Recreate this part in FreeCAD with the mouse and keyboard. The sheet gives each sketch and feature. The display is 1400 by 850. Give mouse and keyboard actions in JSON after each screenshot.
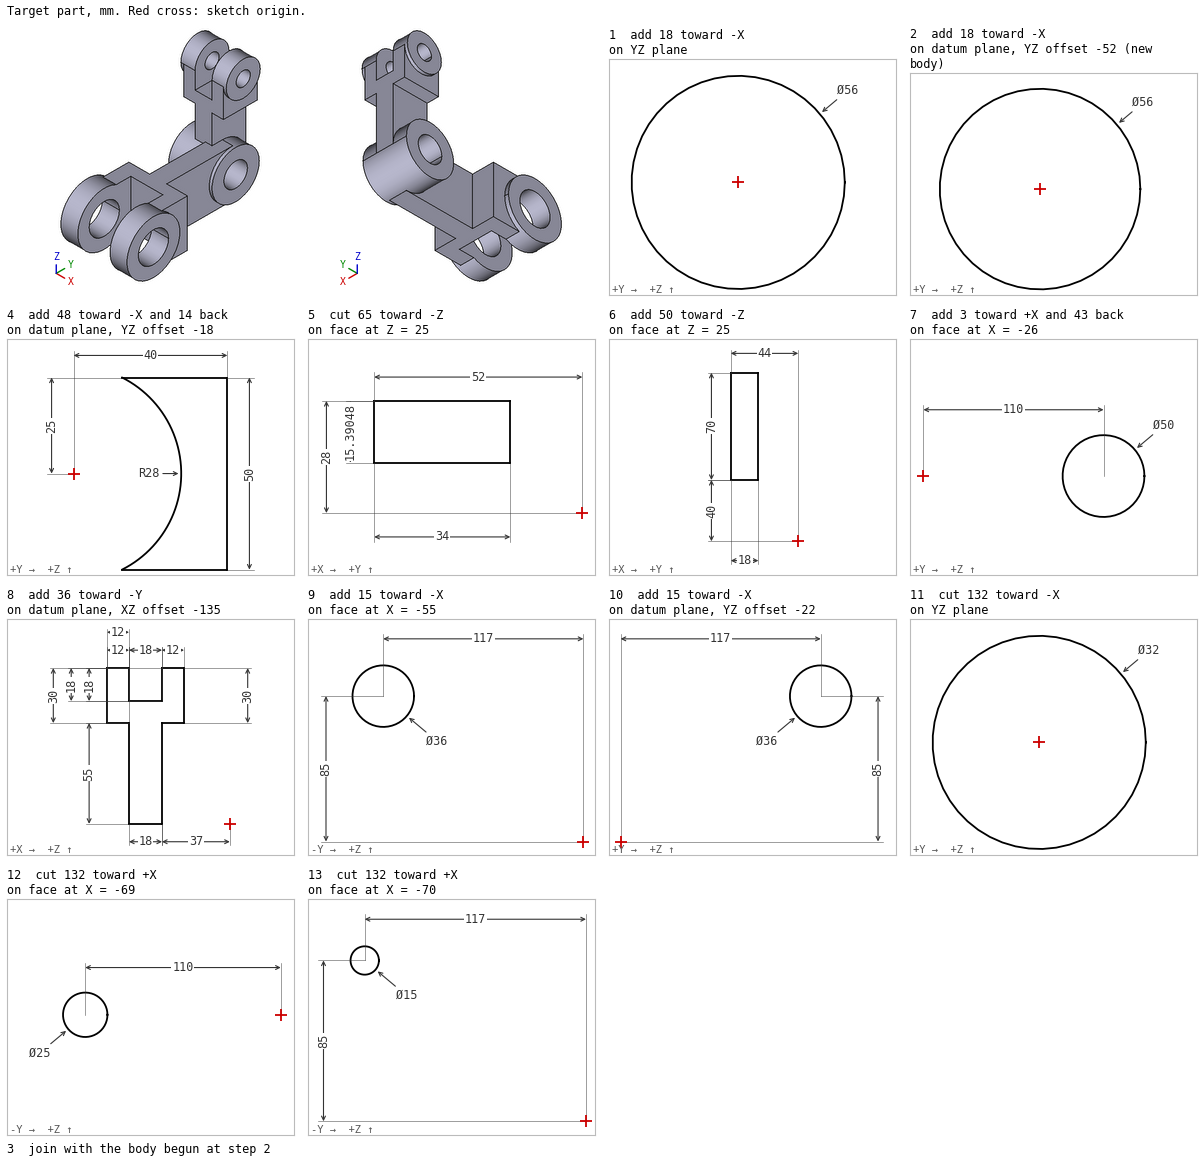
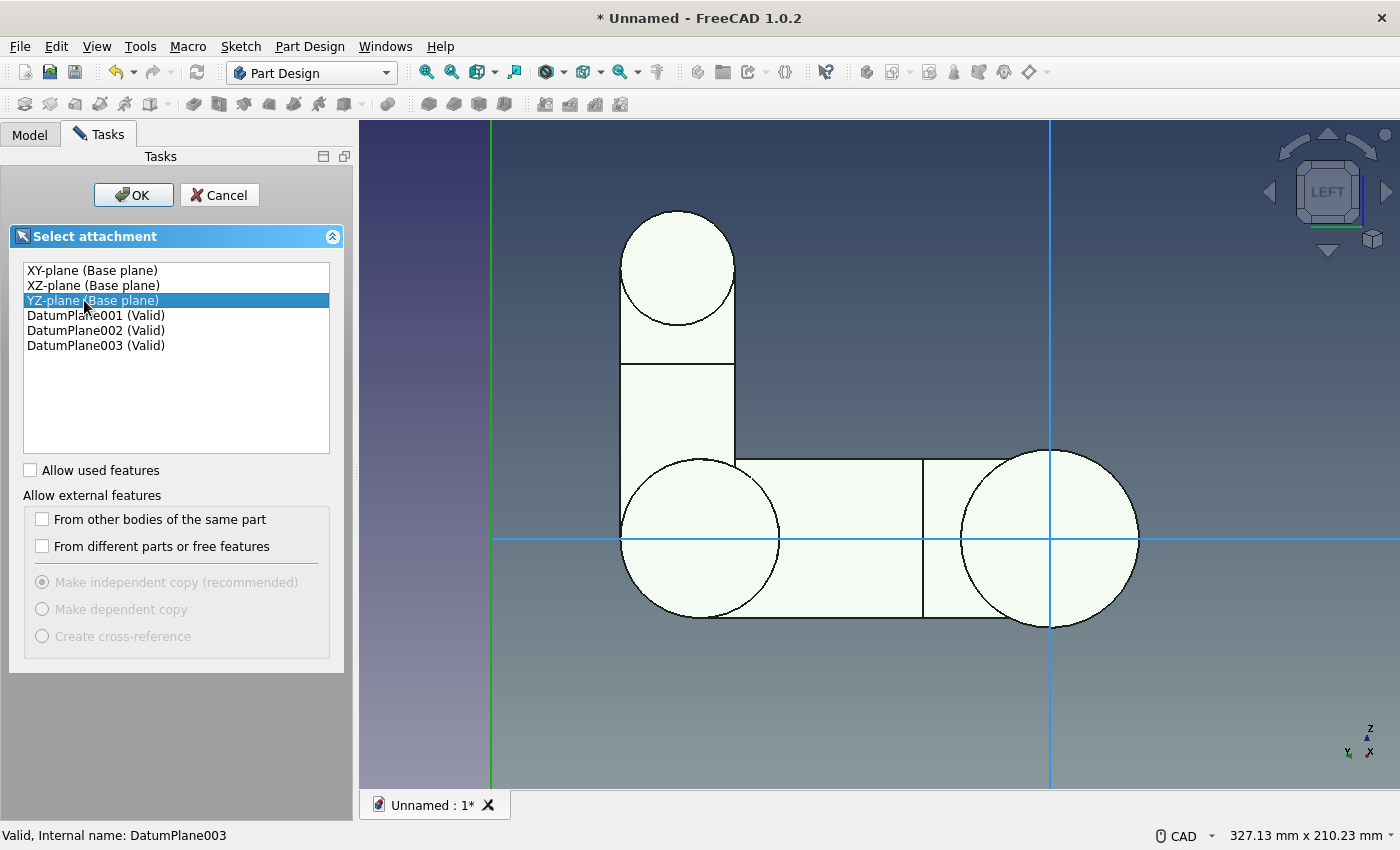
{"action": "left_click", "coordinate": [134, 195]}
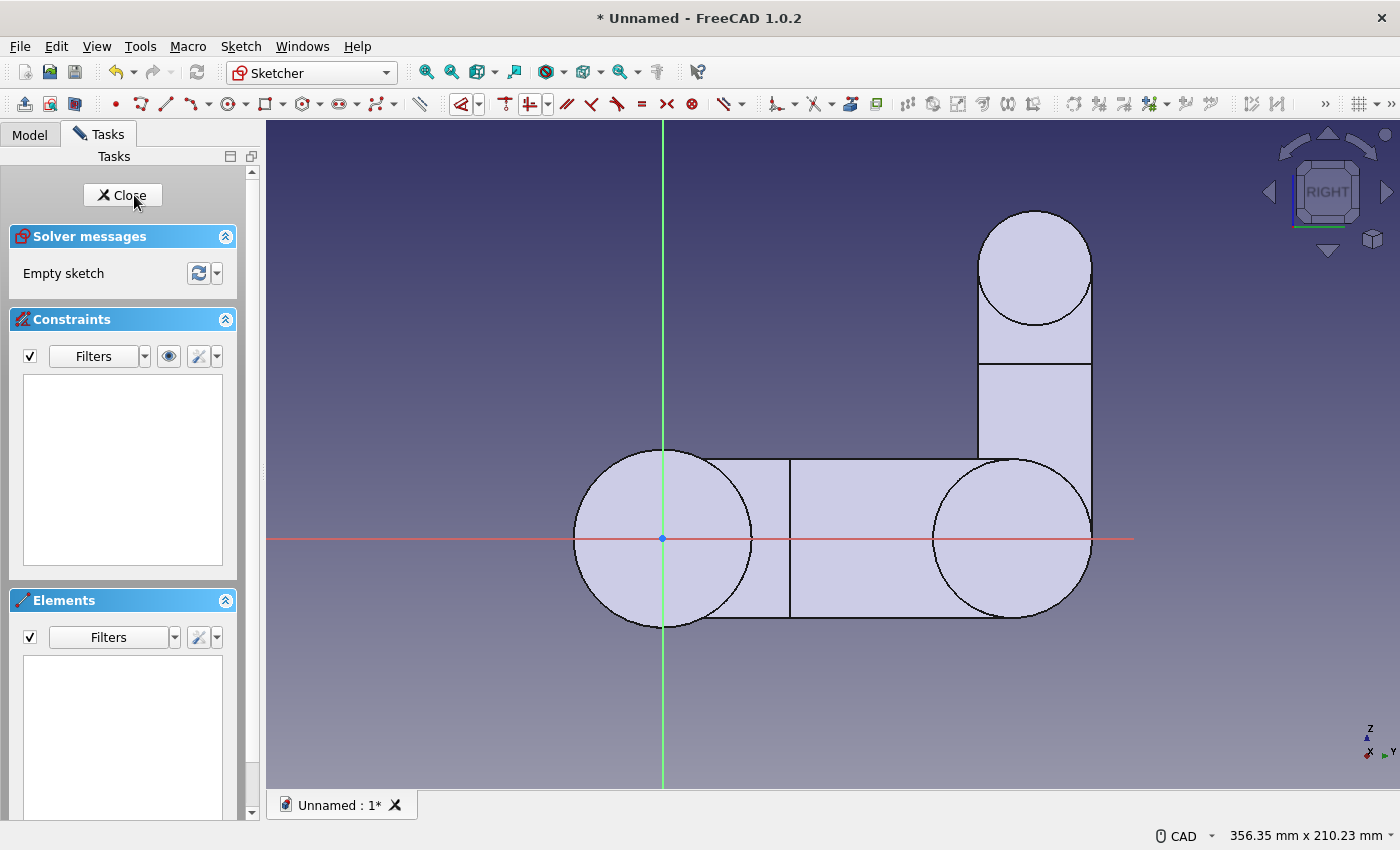
{"action": "scroll", "coordinate": [629, 566], "scroll_direction": "up", "scroll_amount": 7}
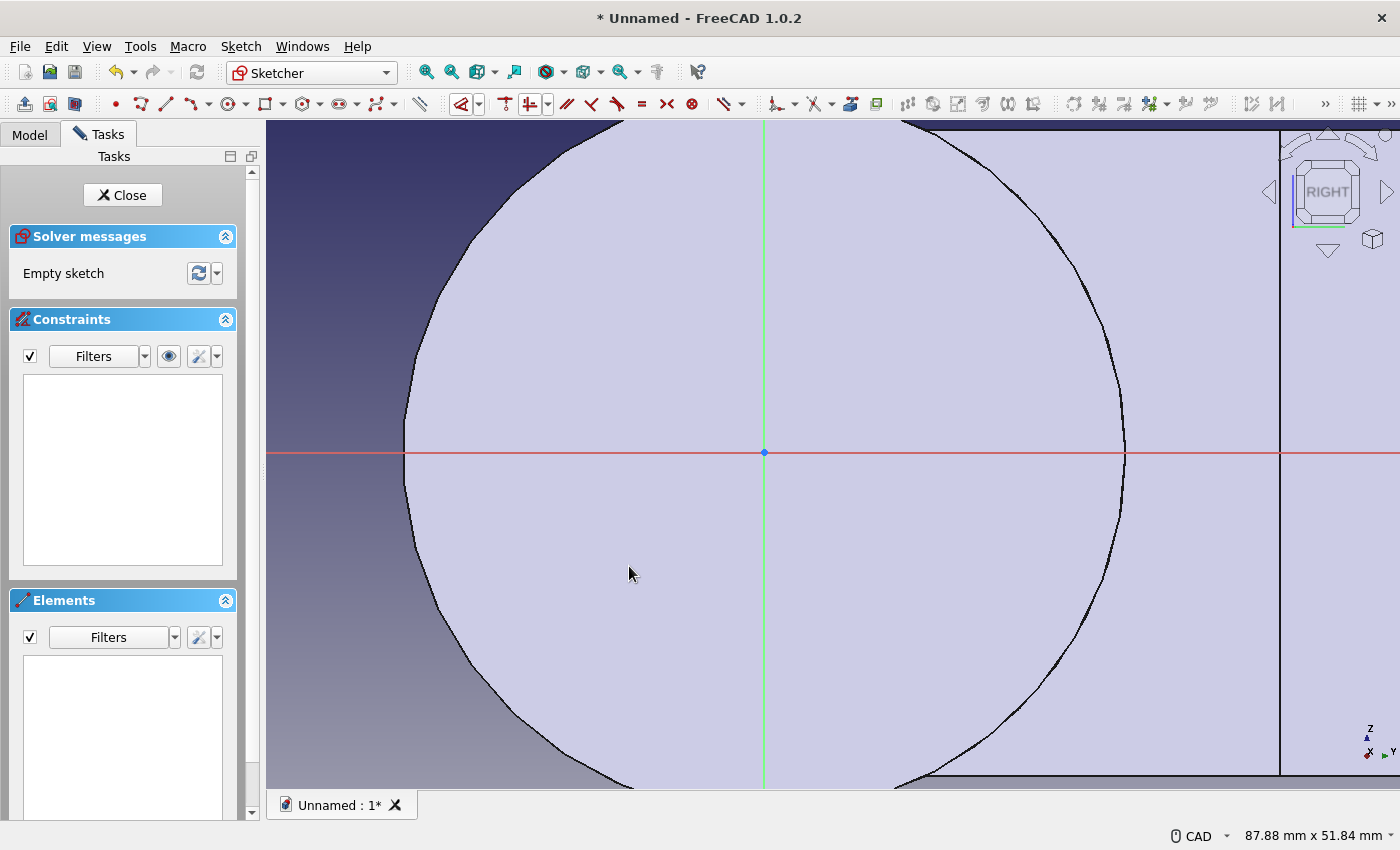
{"action": "key", "text": "g c"}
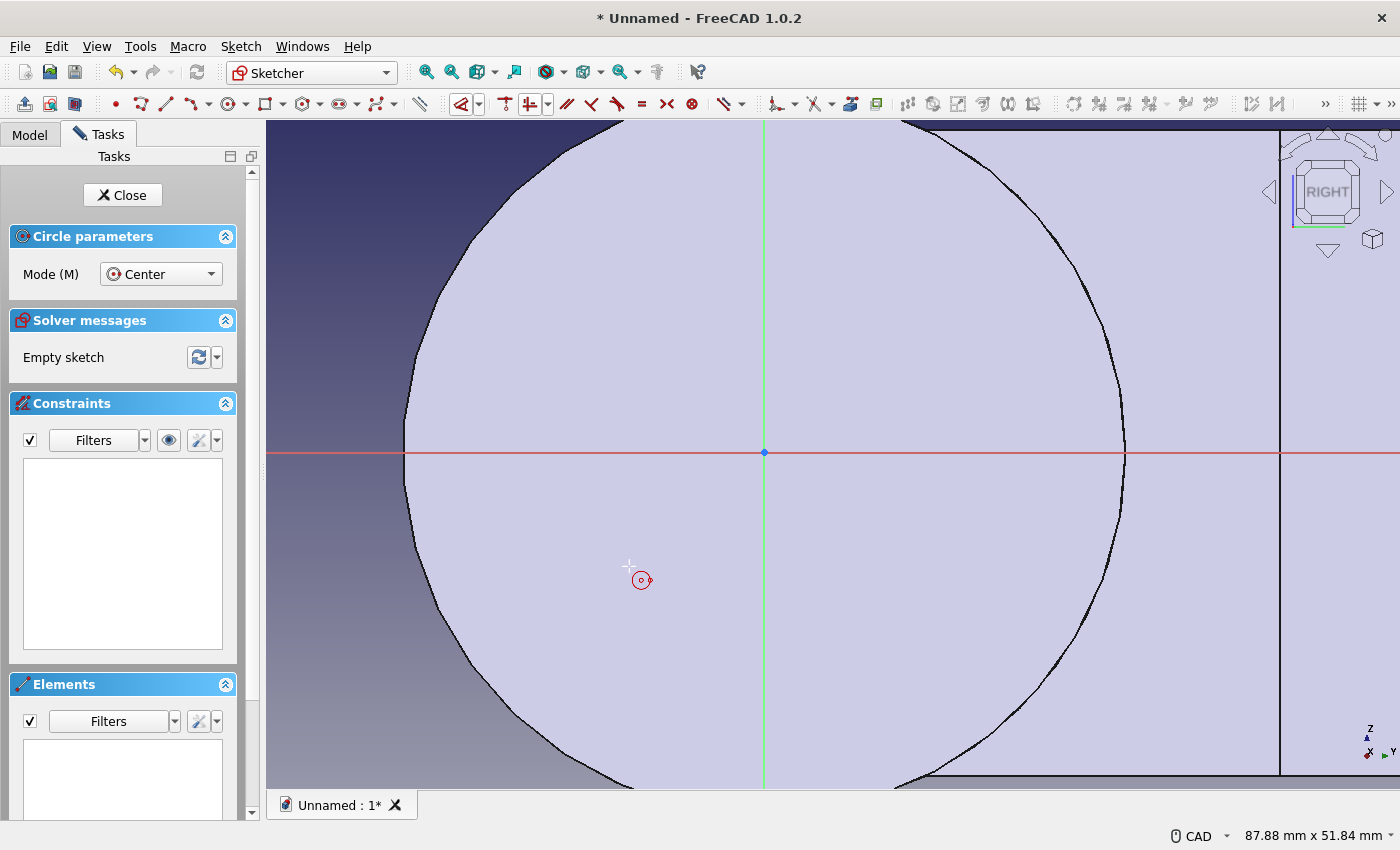
{"action": "left_click", "coordinate": [764, 453]}
{"action": "left_click", "coordinate": [910, 307]}
{"action": "key", "text": "Escape"}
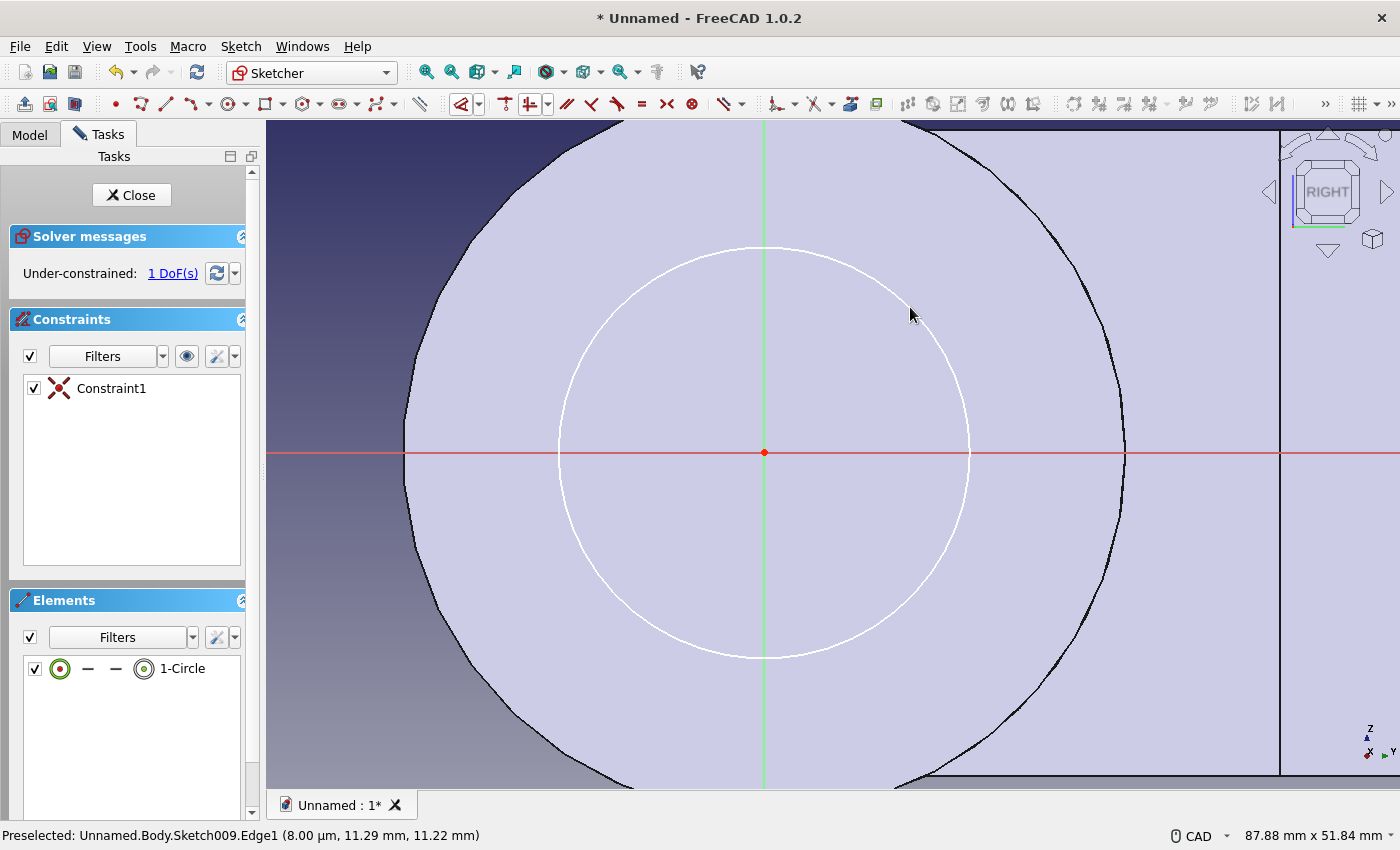
{"action": "left_click", "coordinate": [909, 307]}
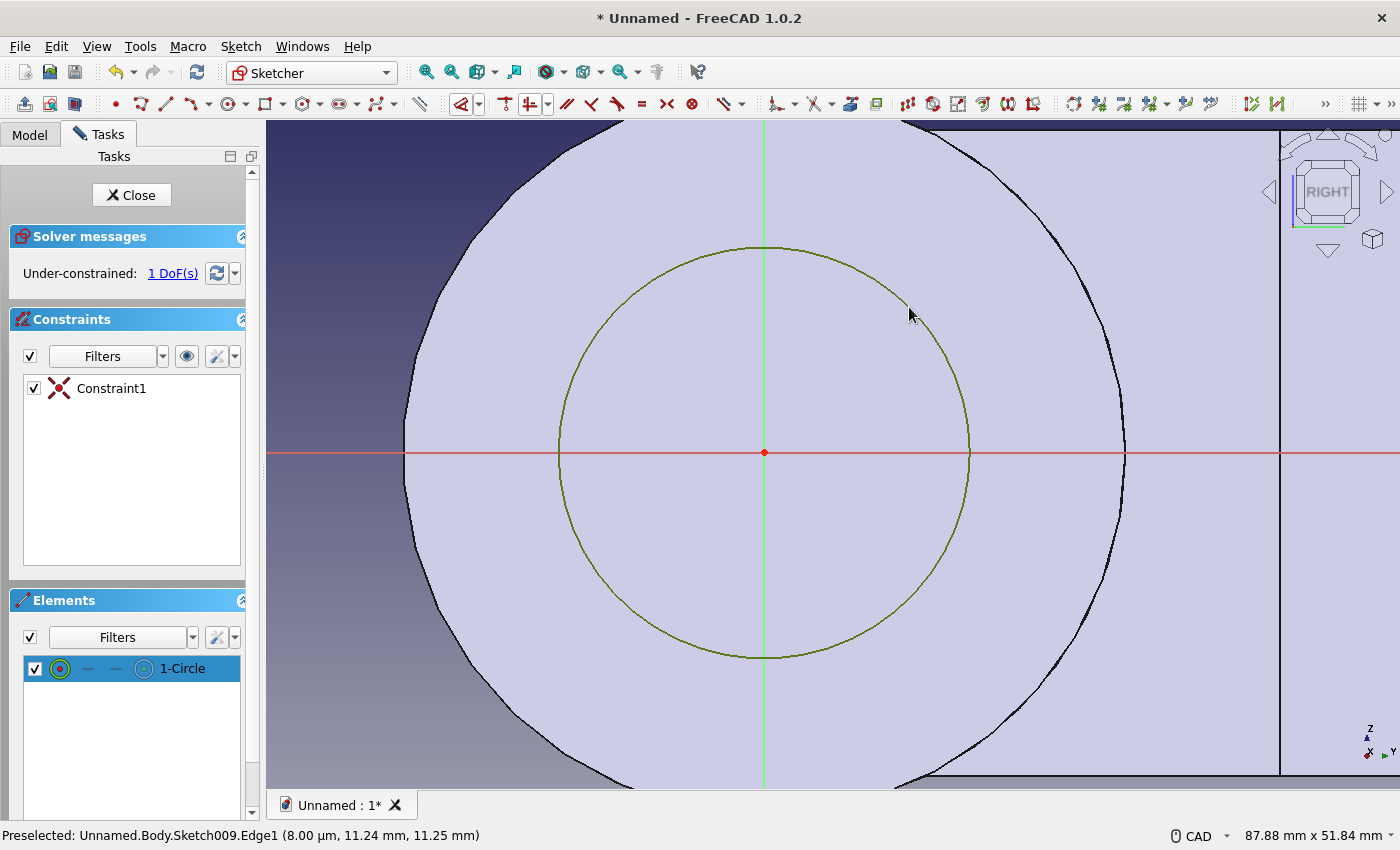
{"action": "left_click", "coordinate": [478, 104]}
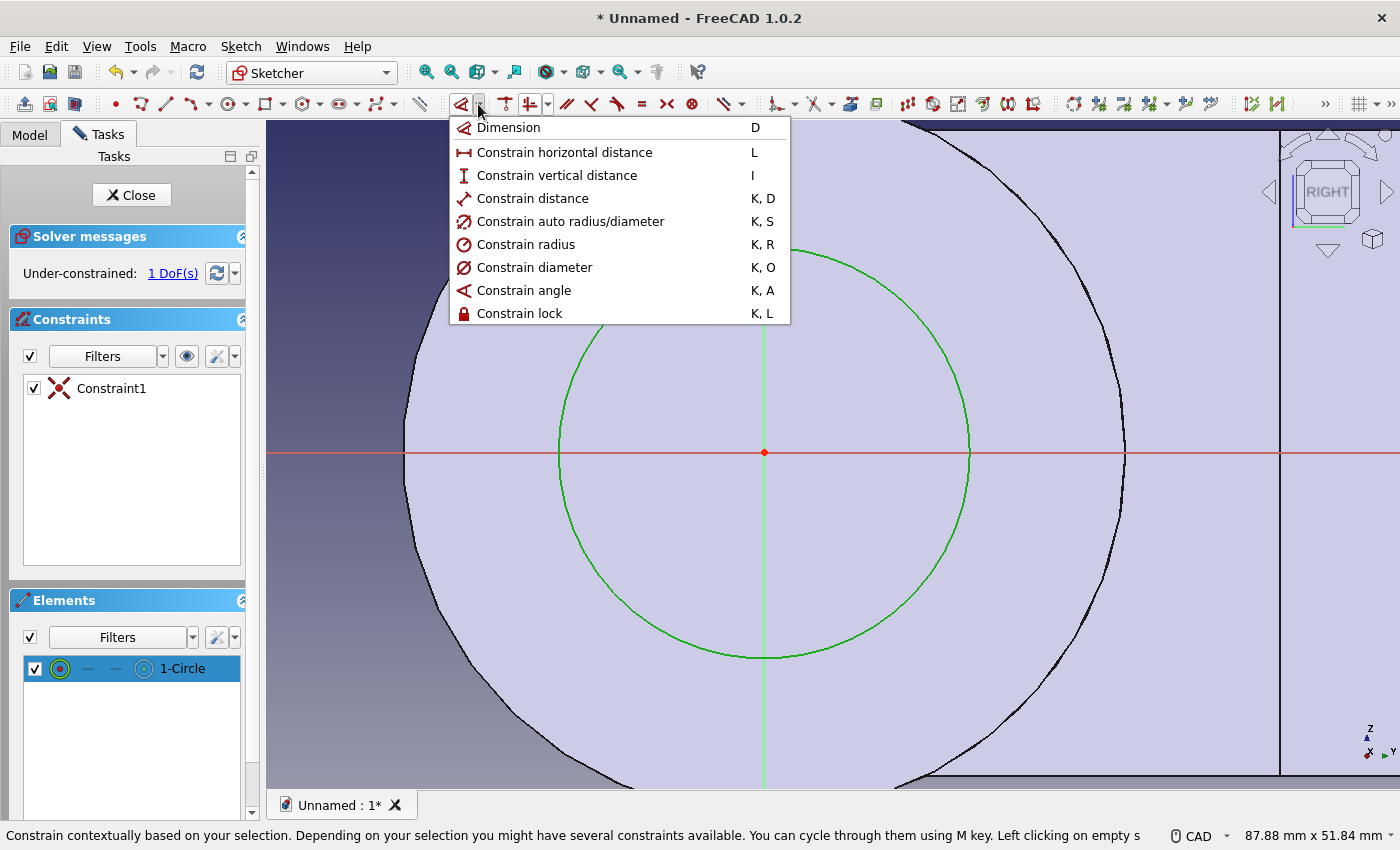
{"action": "left_click", "coordinate": [620, 268]}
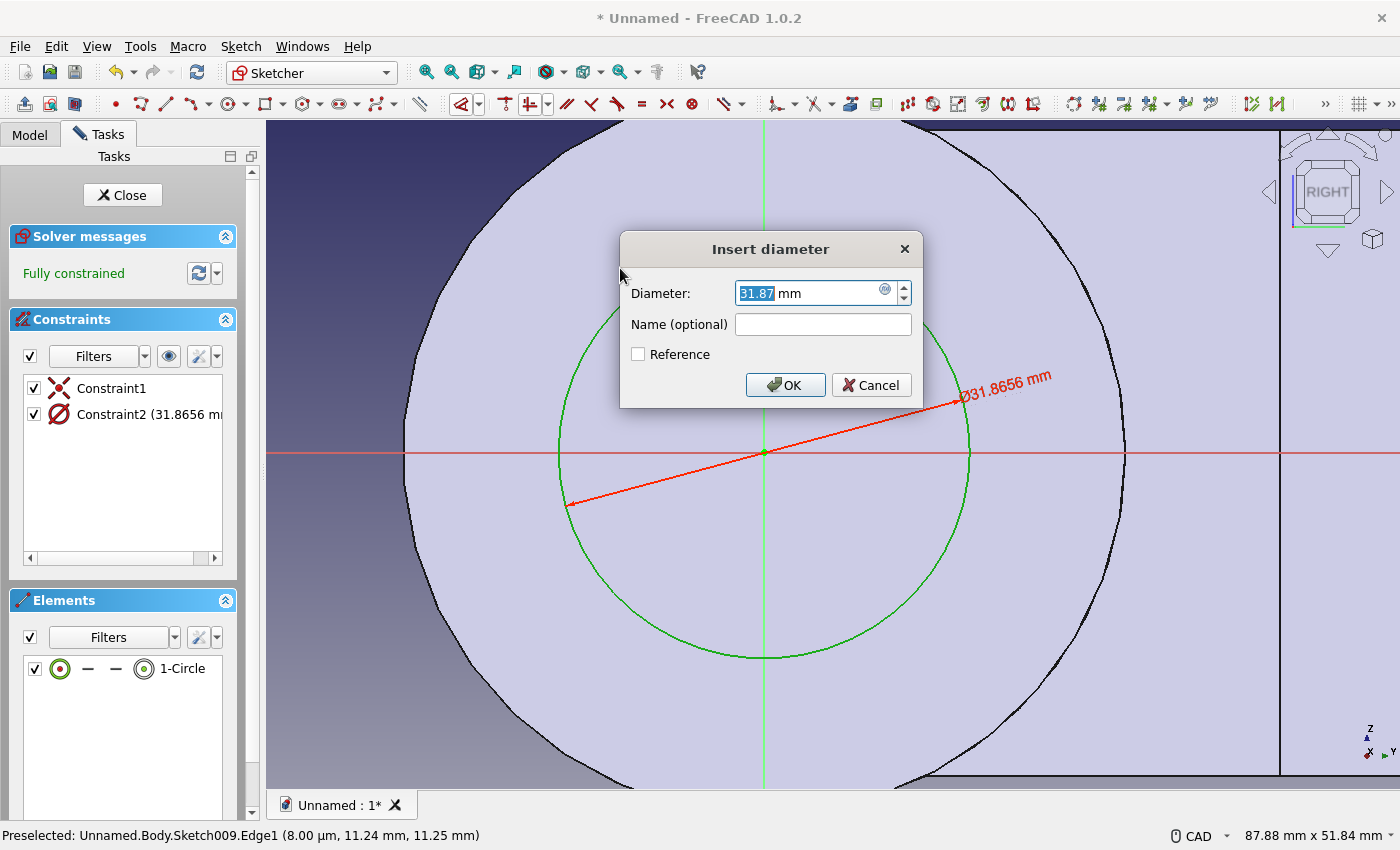
{"action": "type", "text": "32"}
{"action": "key", "text": "Return"}